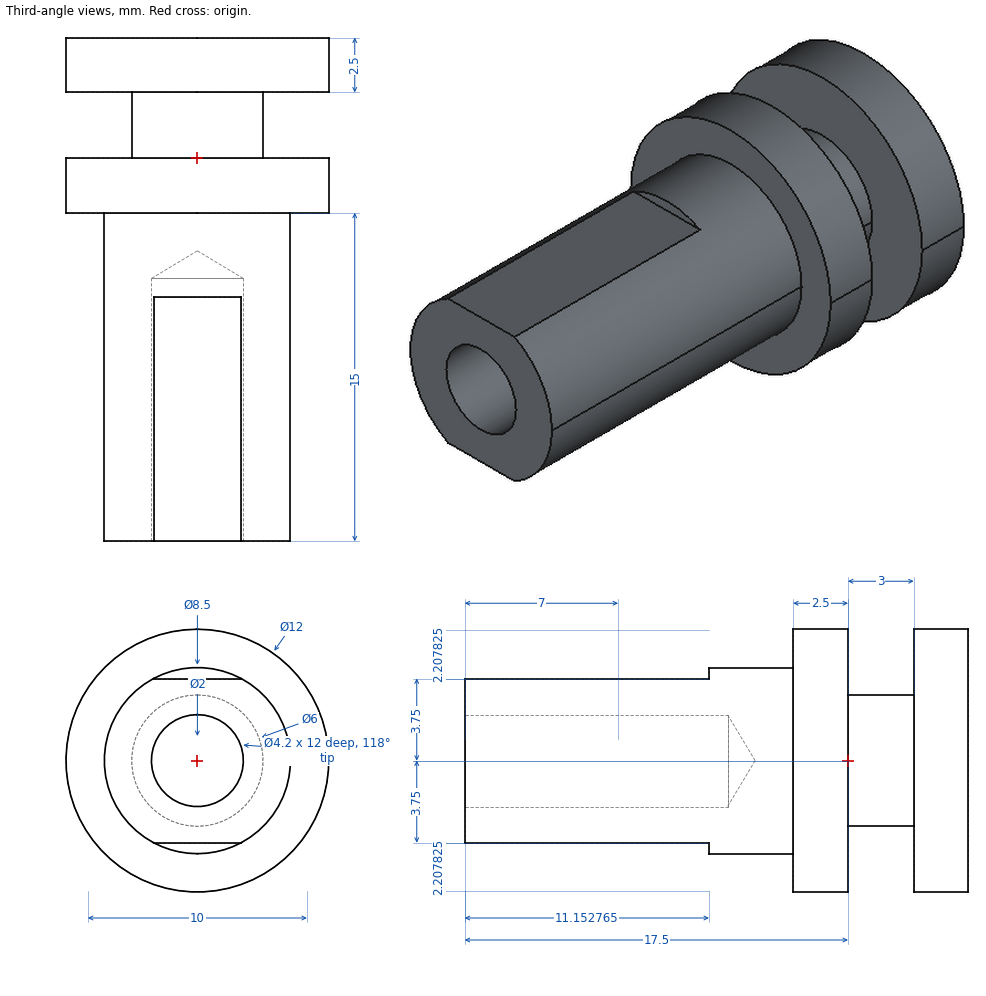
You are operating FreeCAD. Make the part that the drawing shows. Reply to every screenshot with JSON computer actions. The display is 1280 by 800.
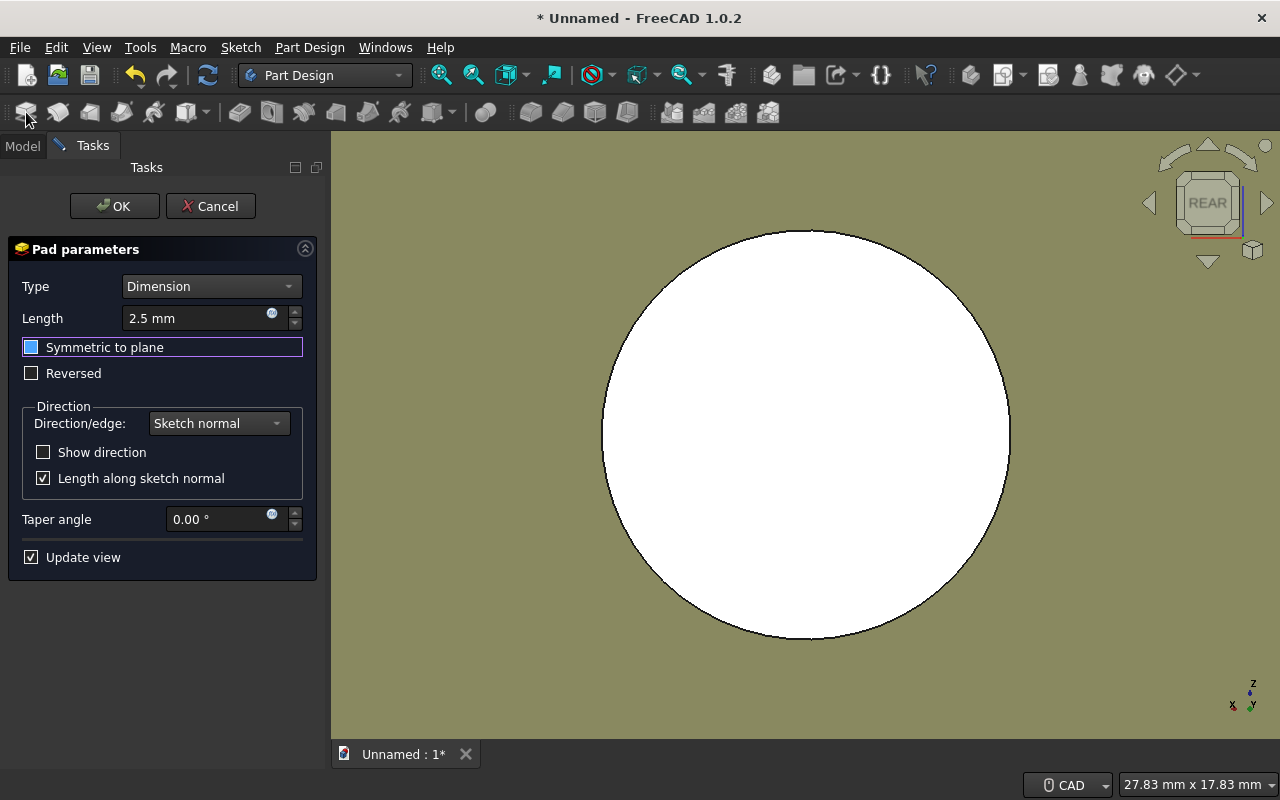
{"action": "left_click", "coordinate": [30, 373]}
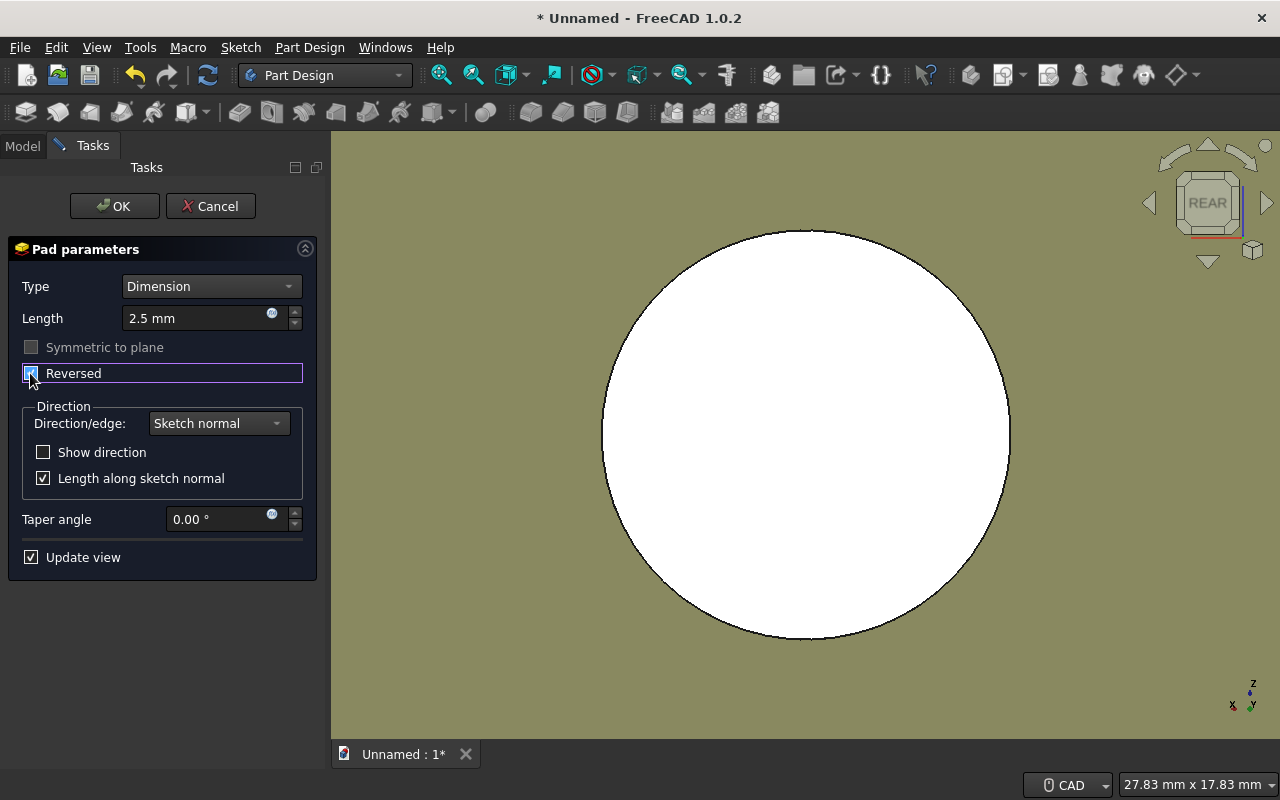
{"action": "left_click", "coordinate": [115, 206]}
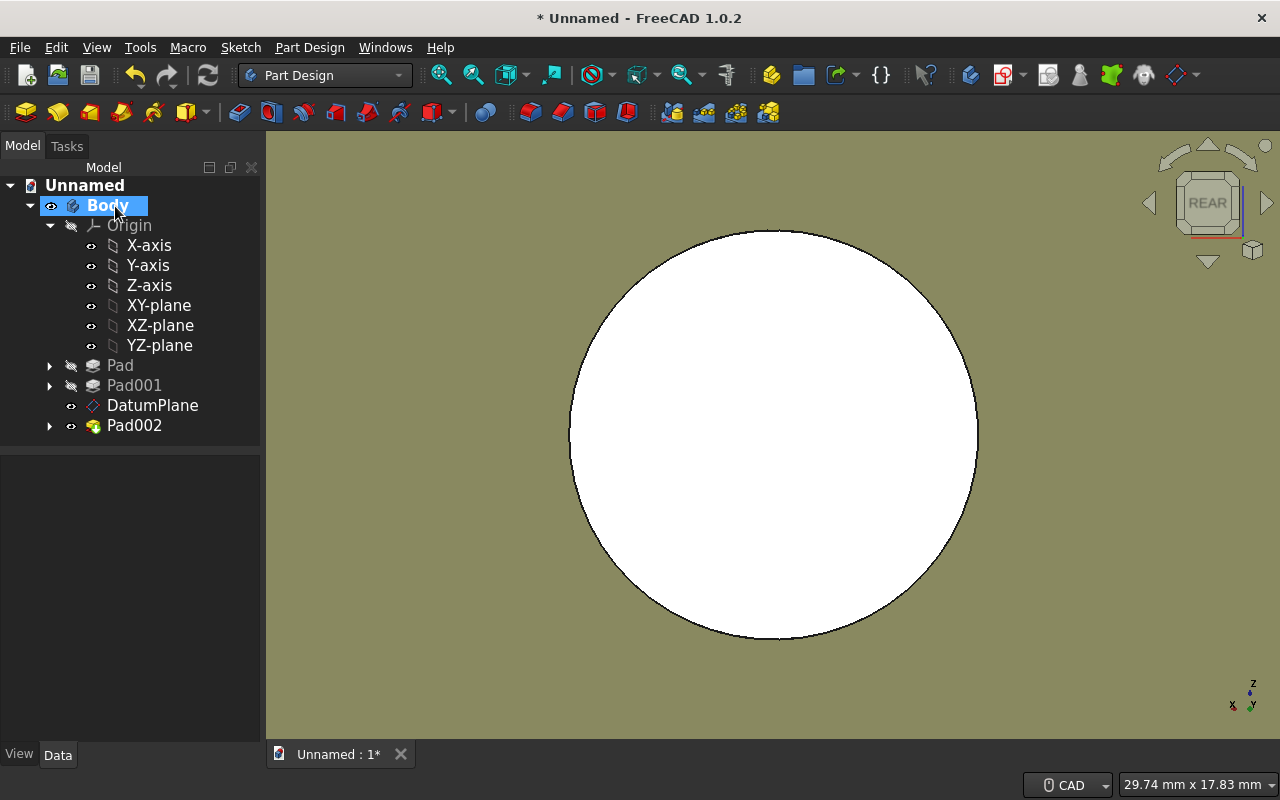
{"action": "left_click", "coordinate": [116, 406]}
{"action": "key", "text": "space"}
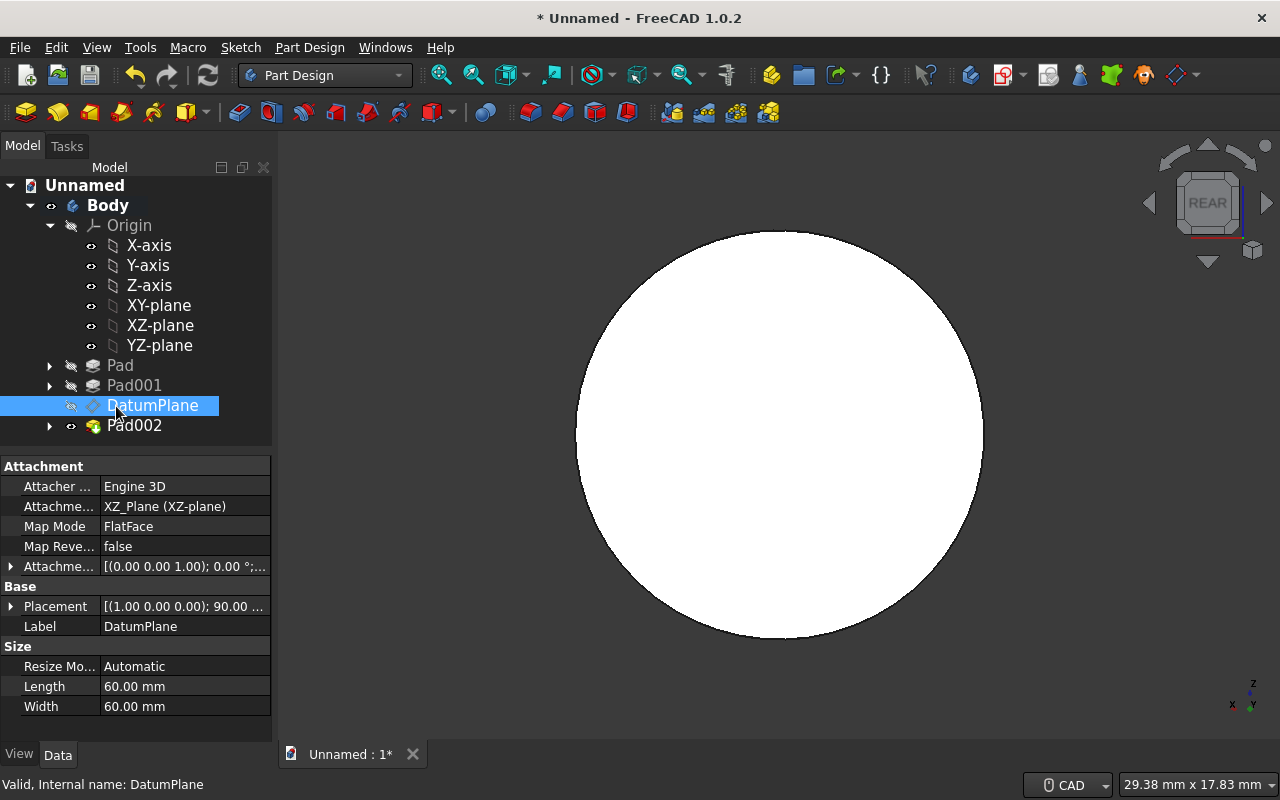
{"action": "key", "text": "0"}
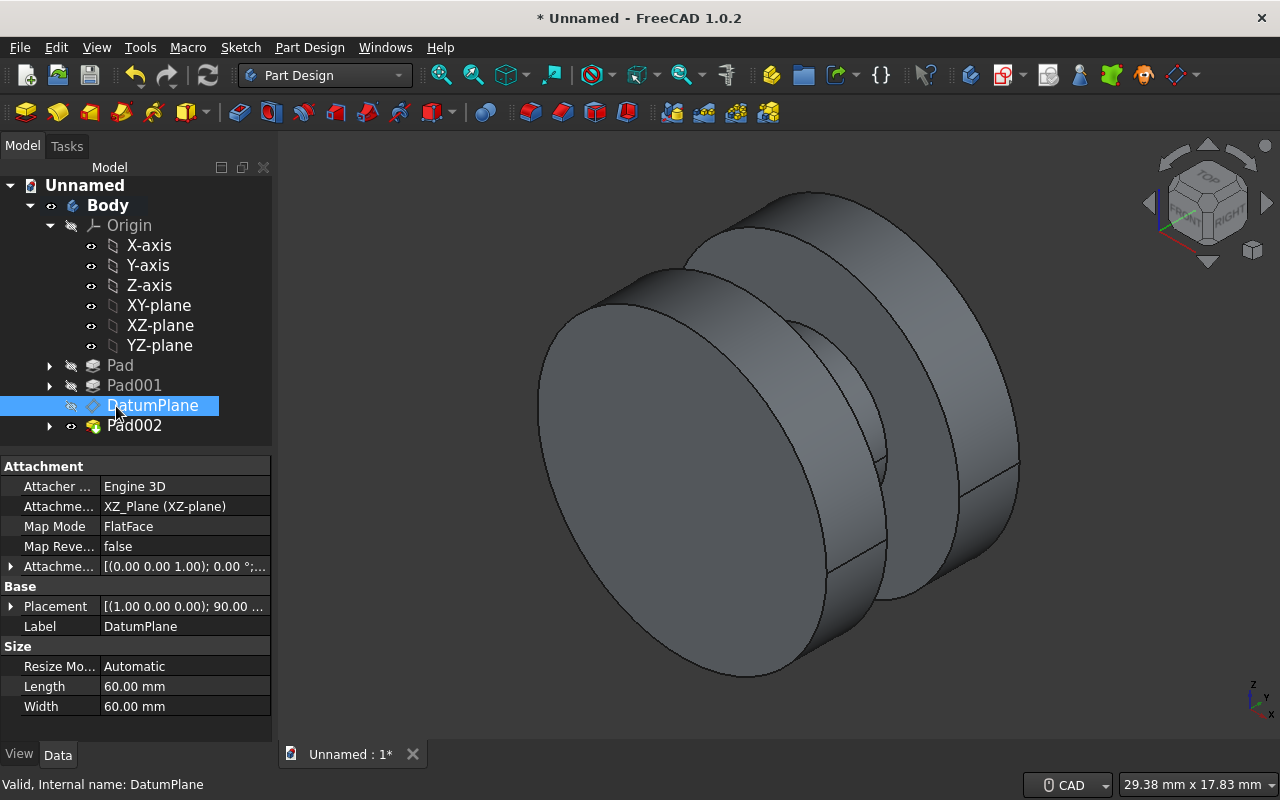
{"action": "key", "text": "v f"}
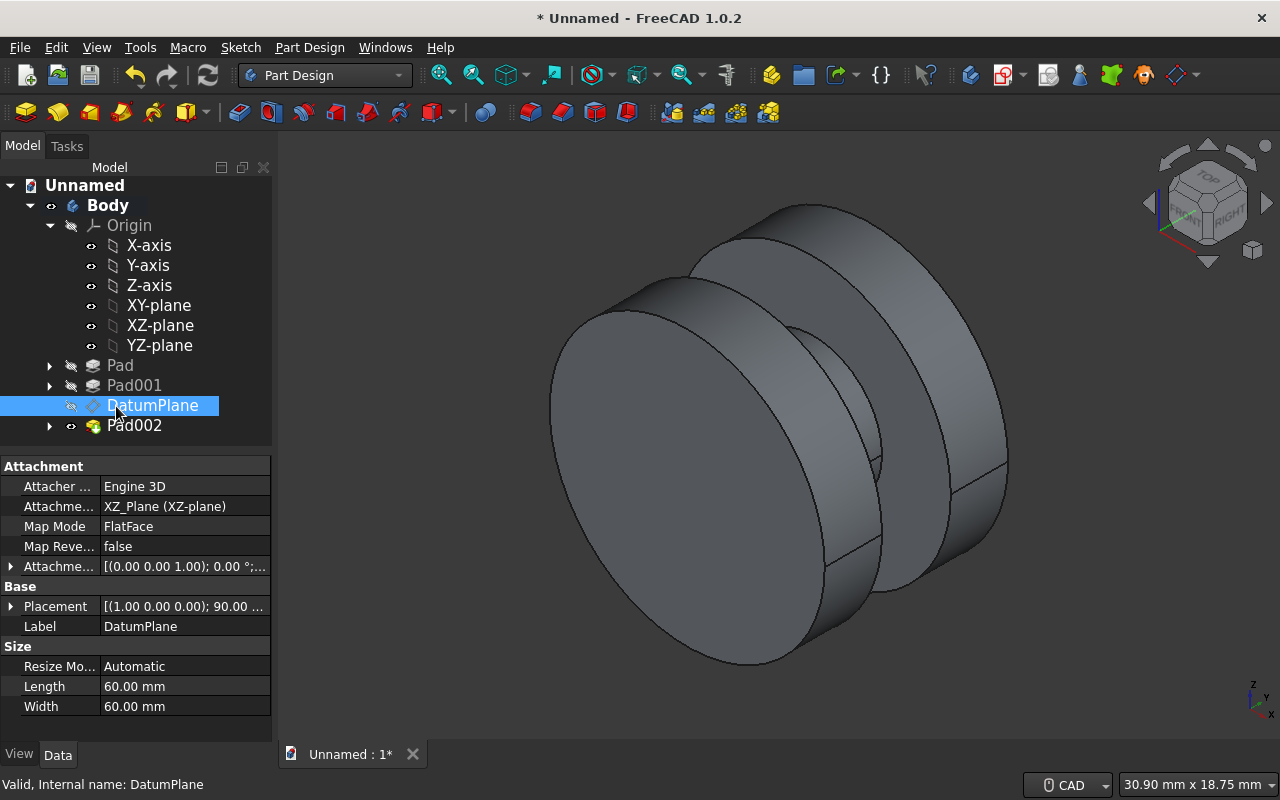
{"action": "left_click", "coordinate": [687, 487]}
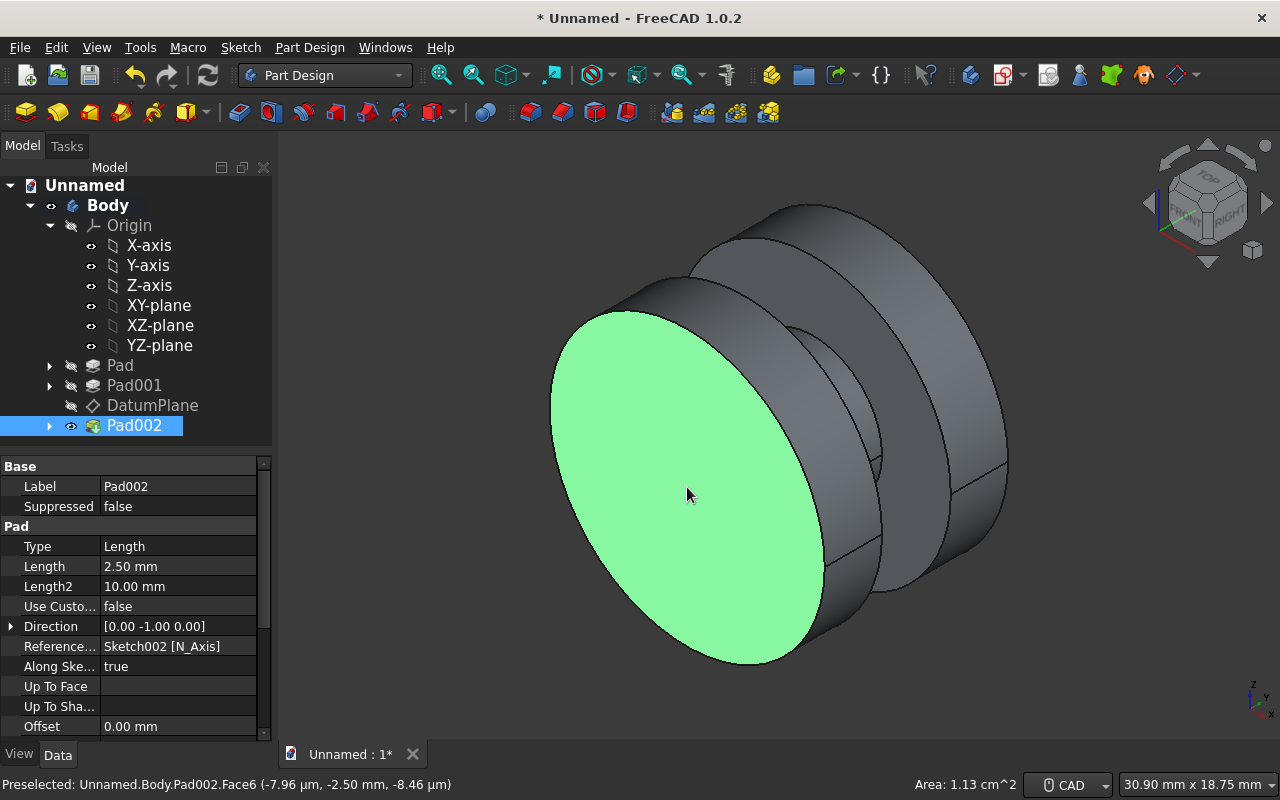
{"action": "left_click", "coordinate": [1004, 76]}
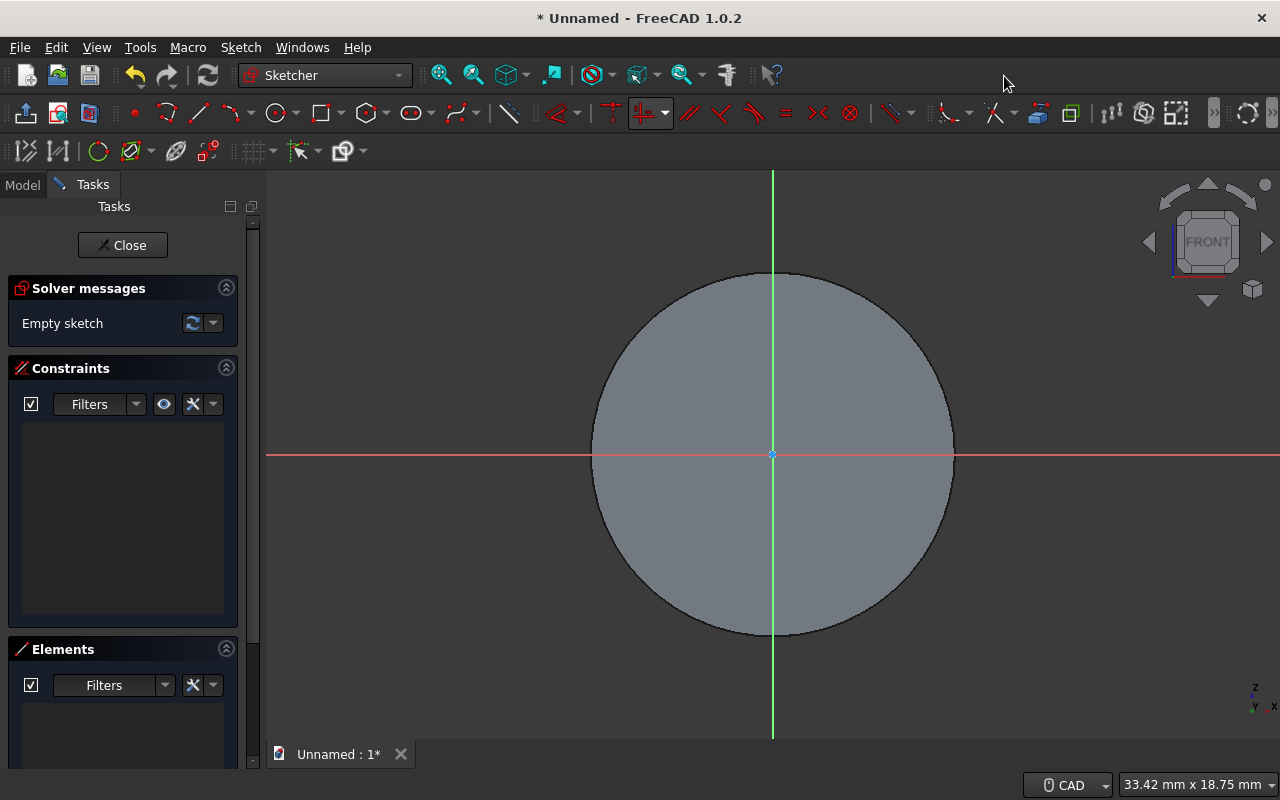
{"action": "scroll", "coordinate": [912, 455], "scroll_direction": "up", "scroll_amount": 2}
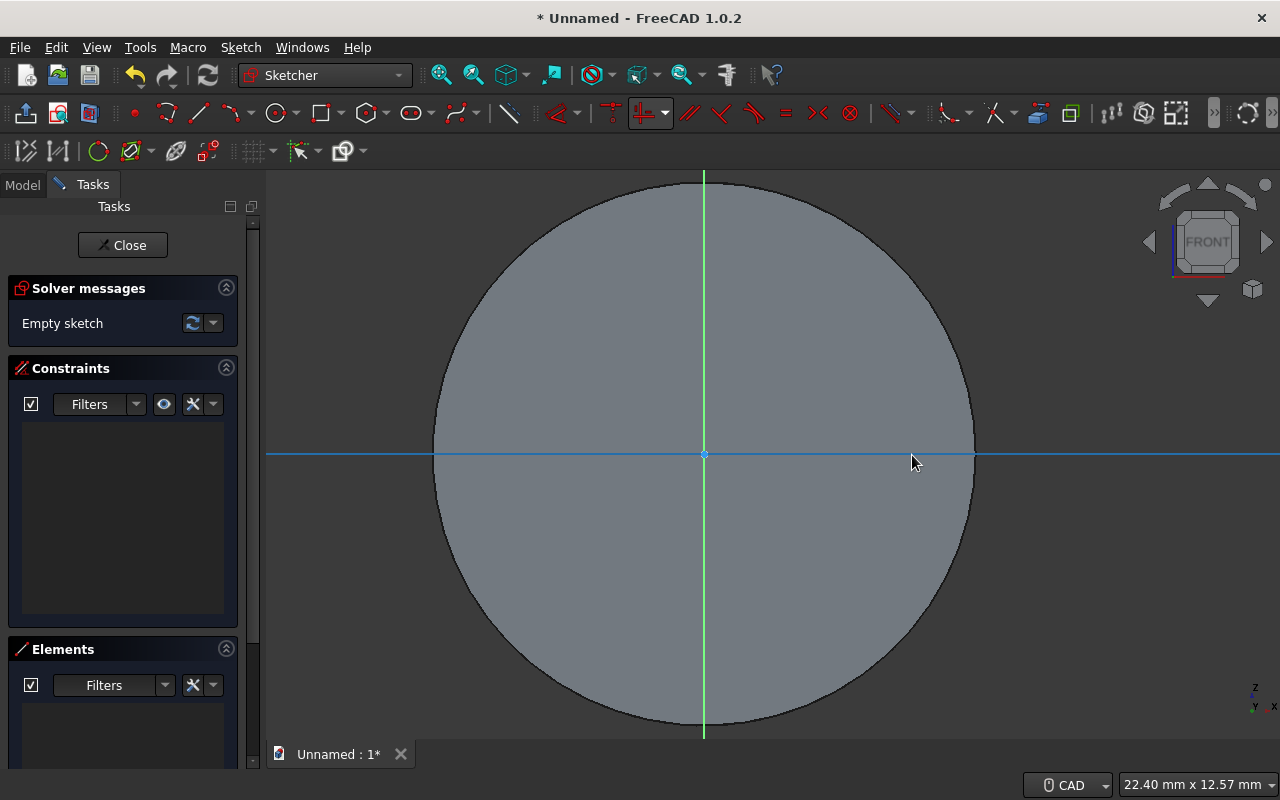
{"action": "left_click", "coordinate": [276, 114]}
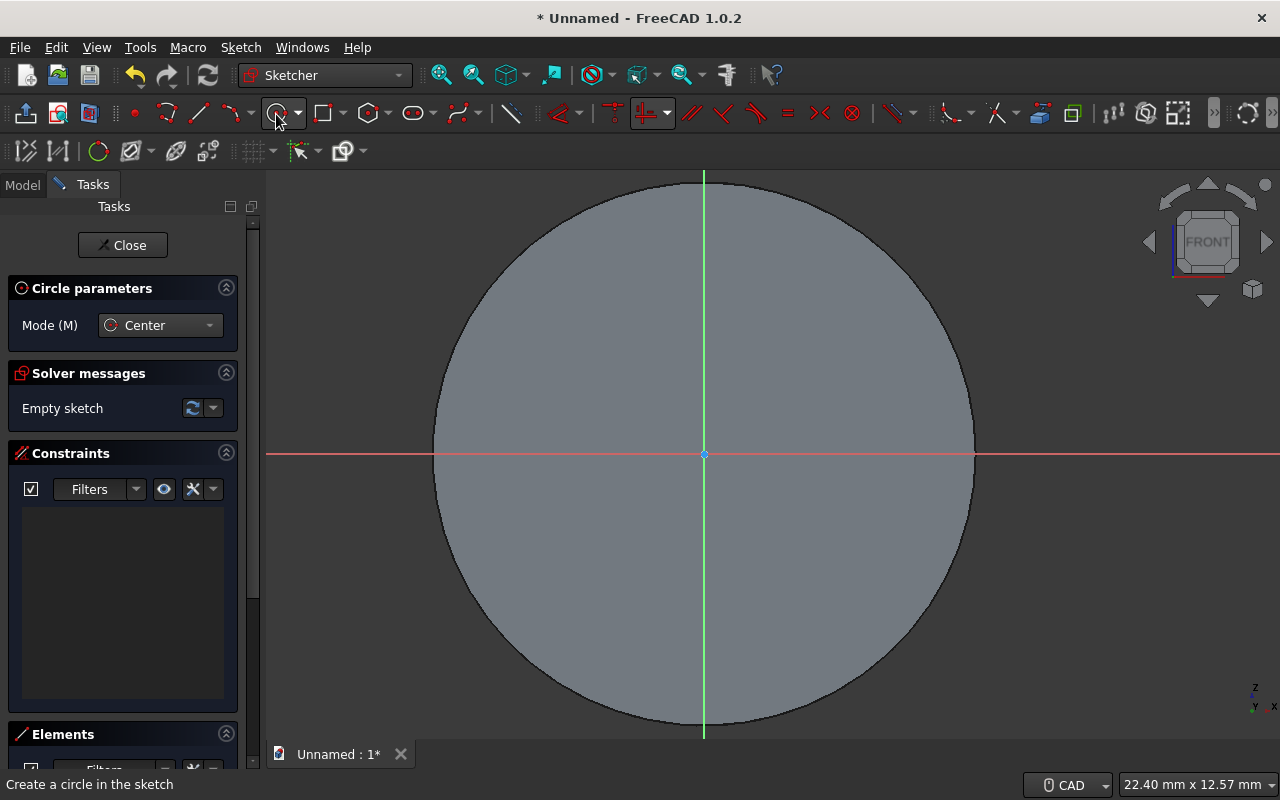
{"action": "left_click", "coordinate": [704, 454]}
{"action": "mouse_move", "coordinate": [840, 318]}